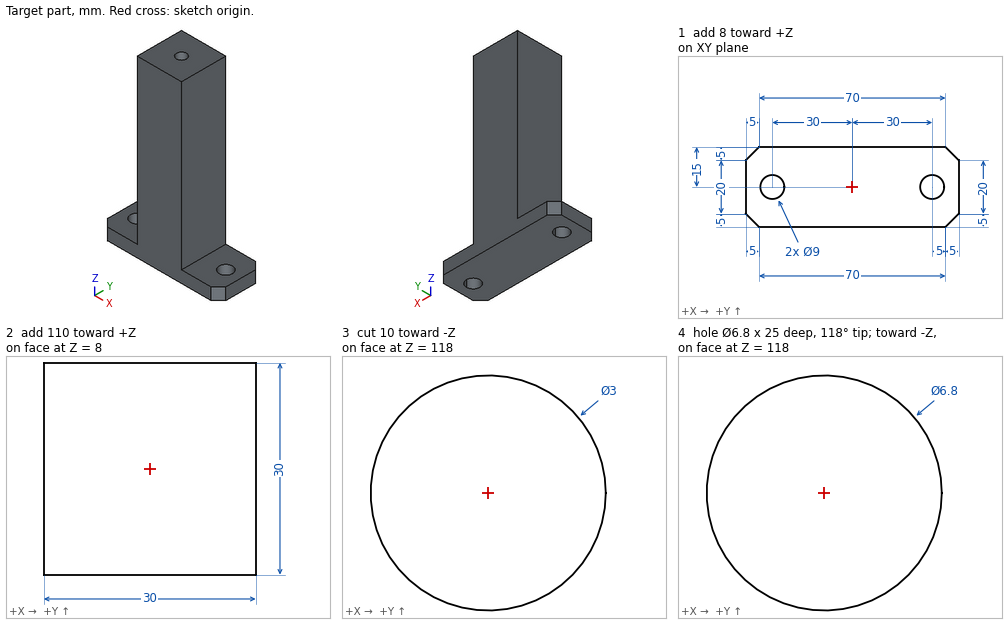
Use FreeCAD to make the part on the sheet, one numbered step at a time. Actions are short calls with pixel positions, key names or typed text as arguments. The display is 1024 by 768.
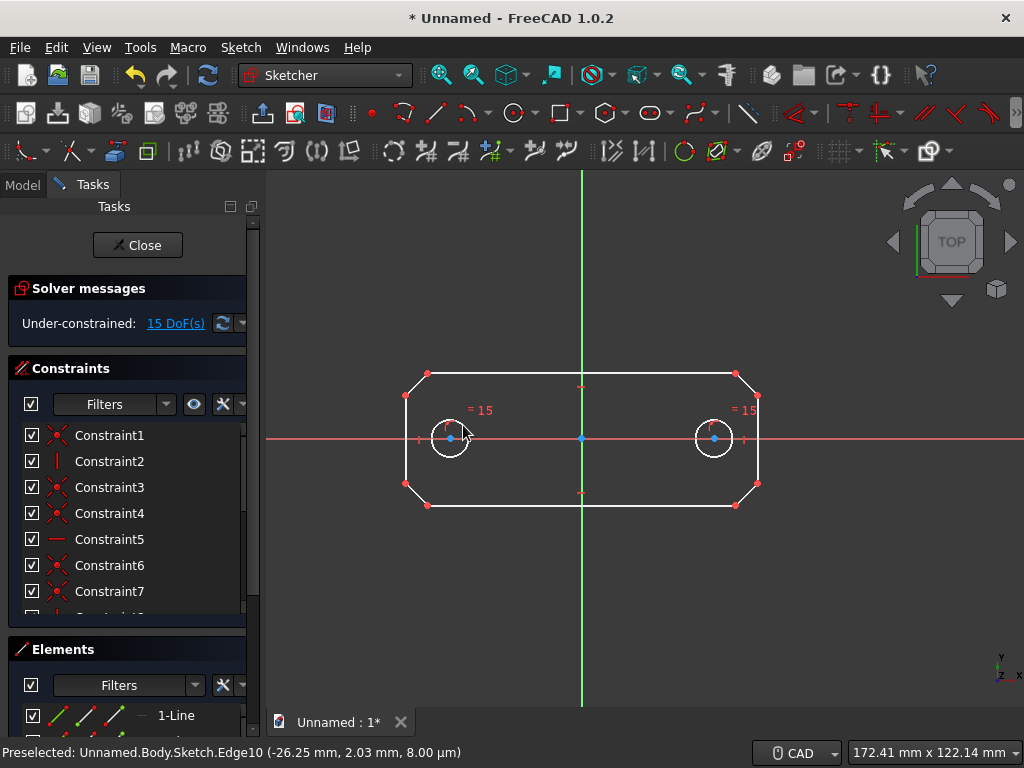
key(d)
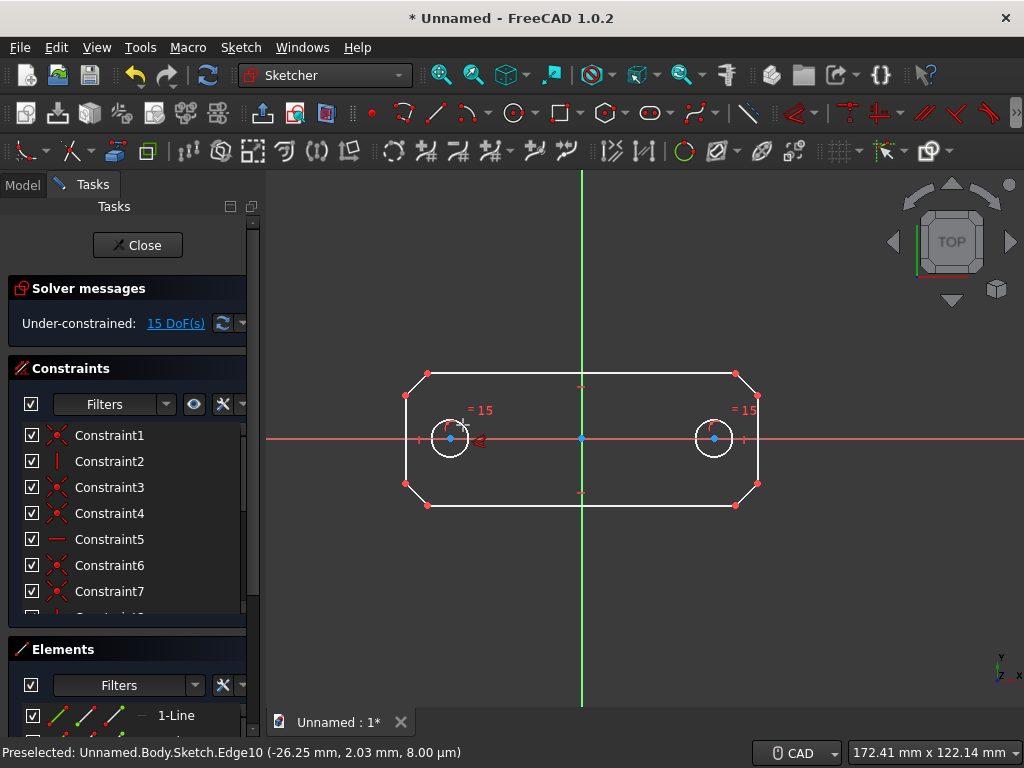
click(727, 425)
click(727, 390)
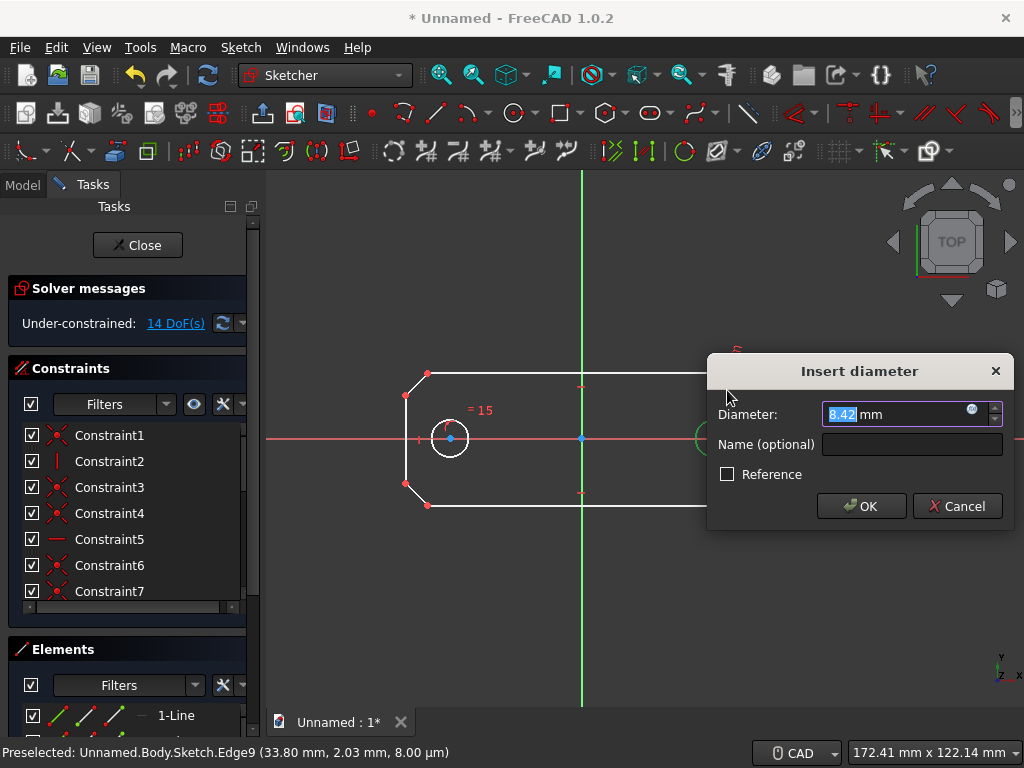
text(9)
key(Return)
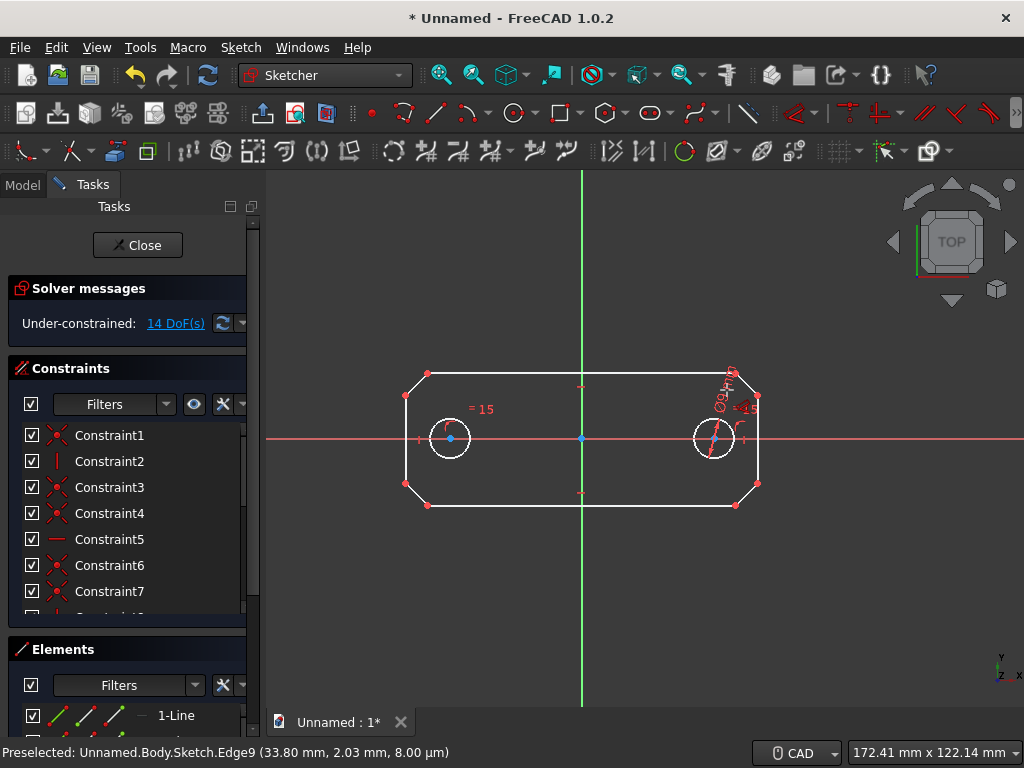
click(406, 422)
click(372, 419)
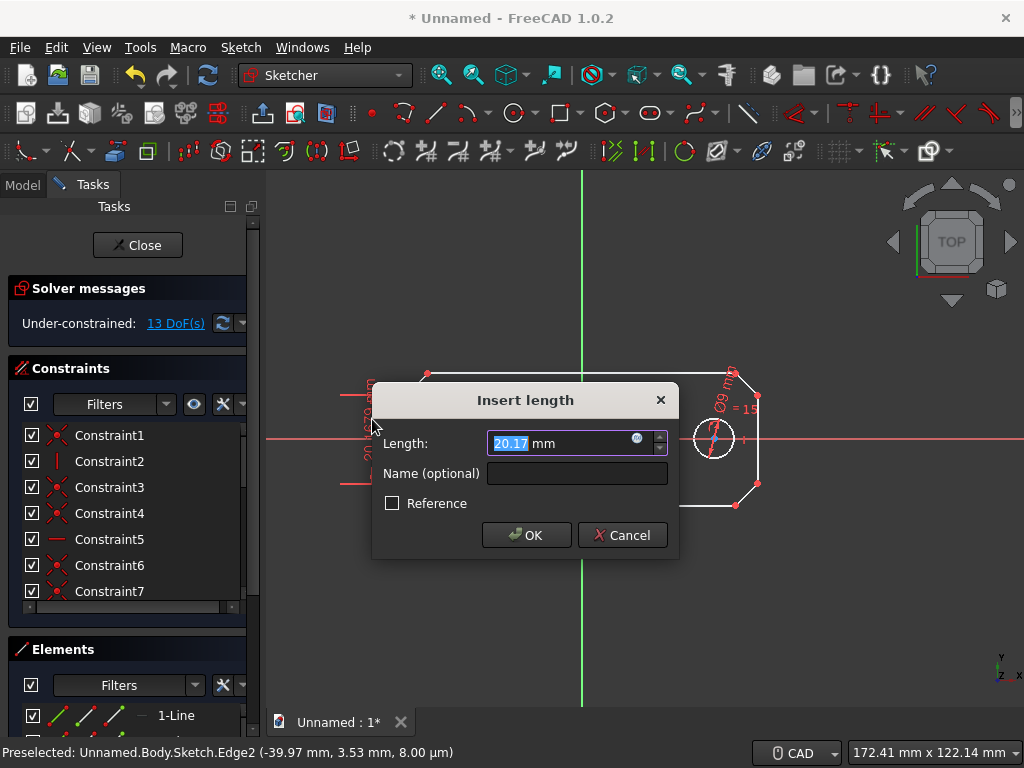
text(20)
key(Return)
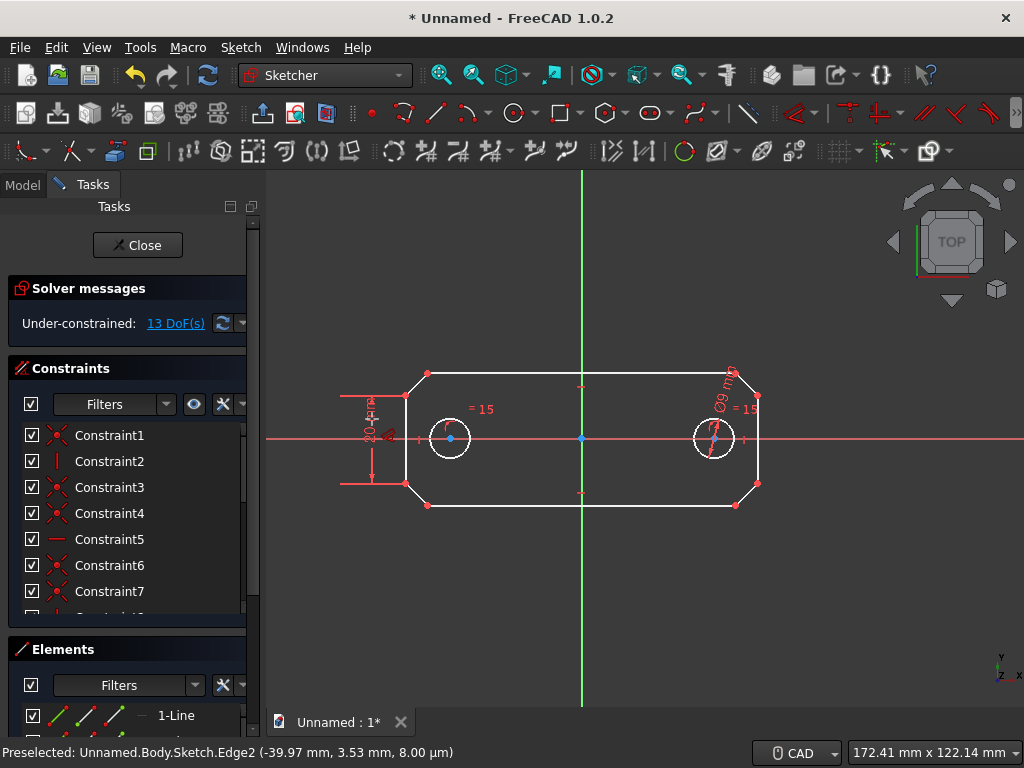
click(520, 506)
click(511, 540)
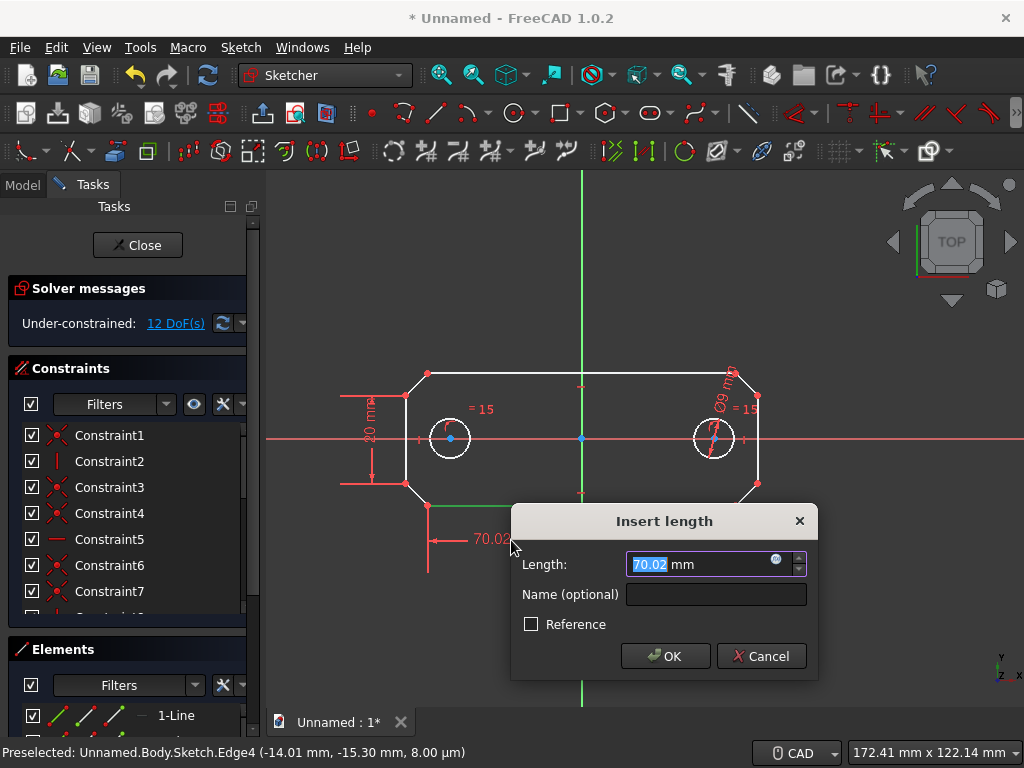
text(70)
key(Return)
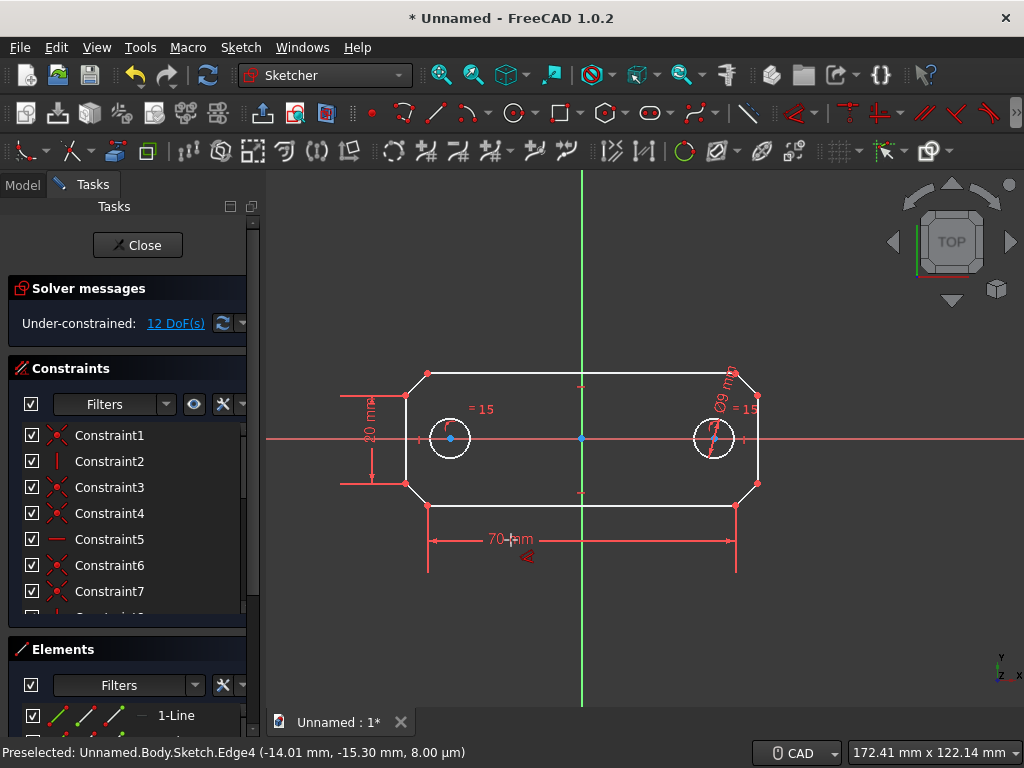
click(758, 457)
click(792, 419)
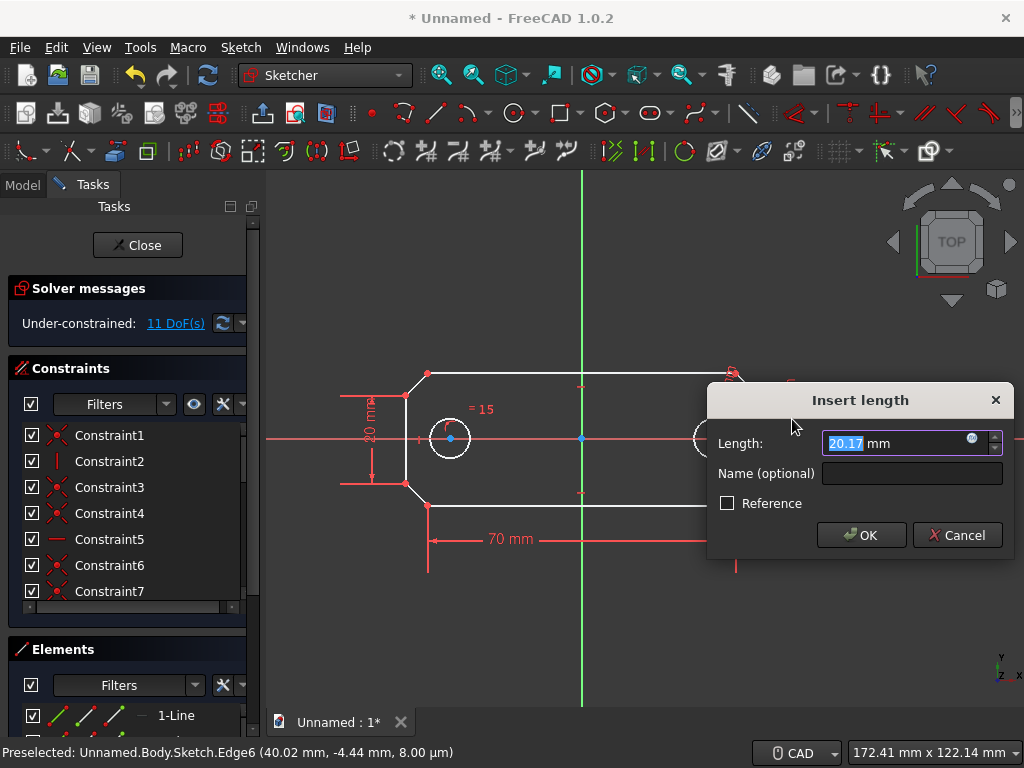
text(20)
key(Return)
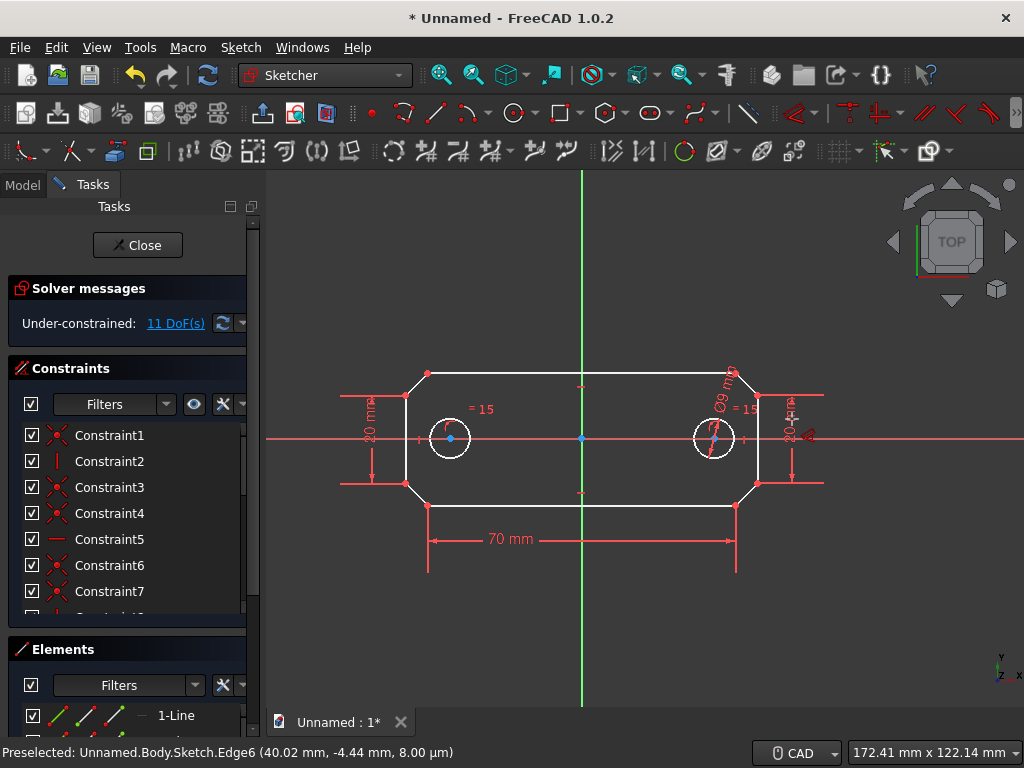
click(643, 373)
click(511, 339)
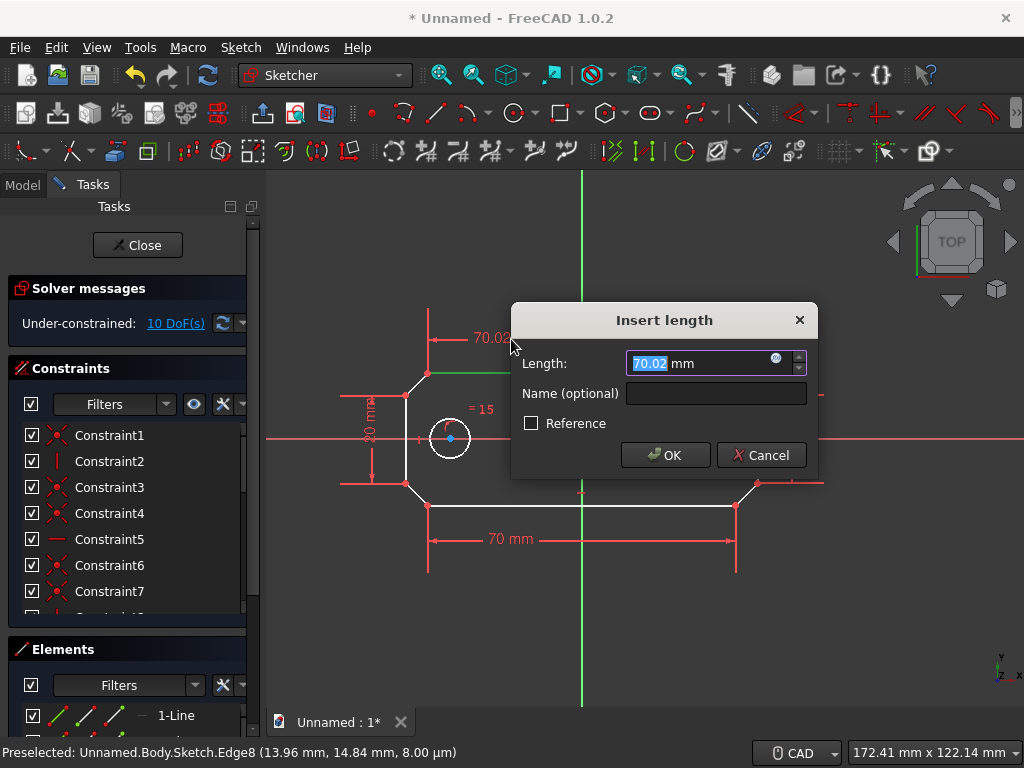
text(70)
key(Return)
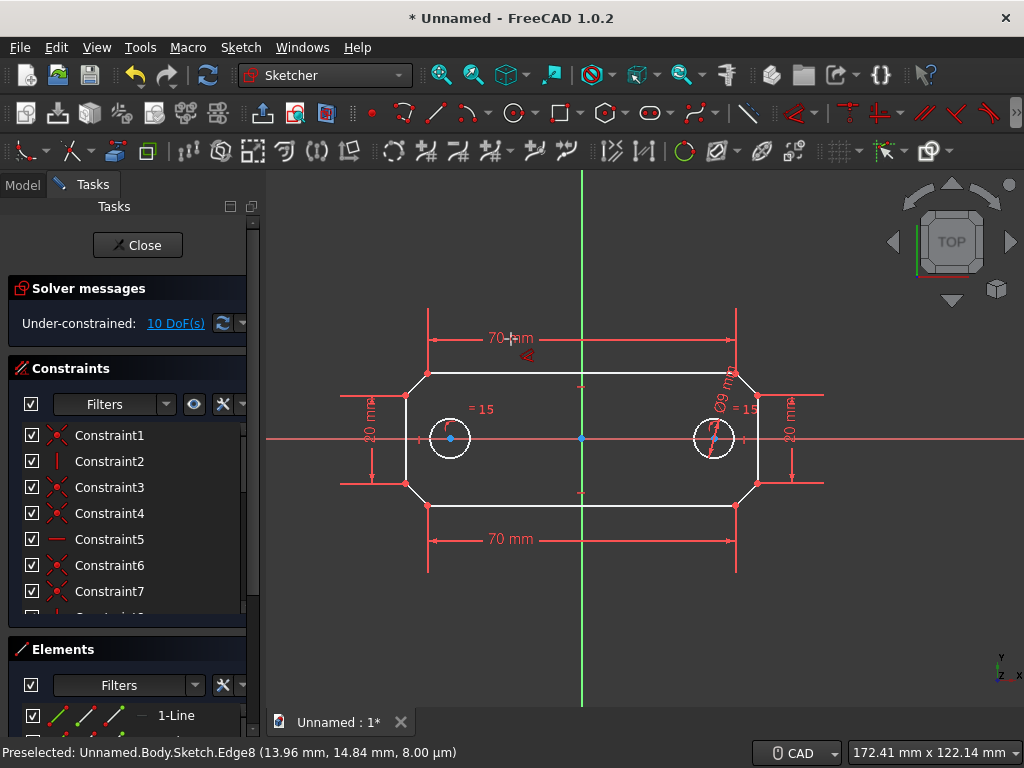
scroll(421, 380, up, 3)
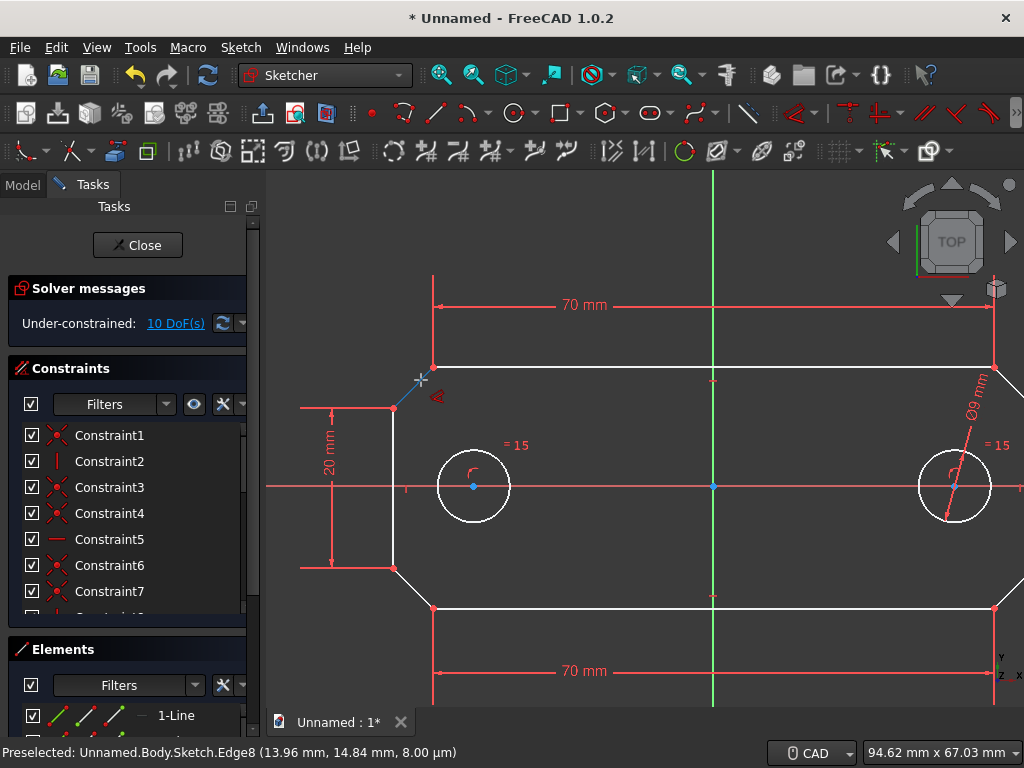
click(421, 380)
click(413, 333)